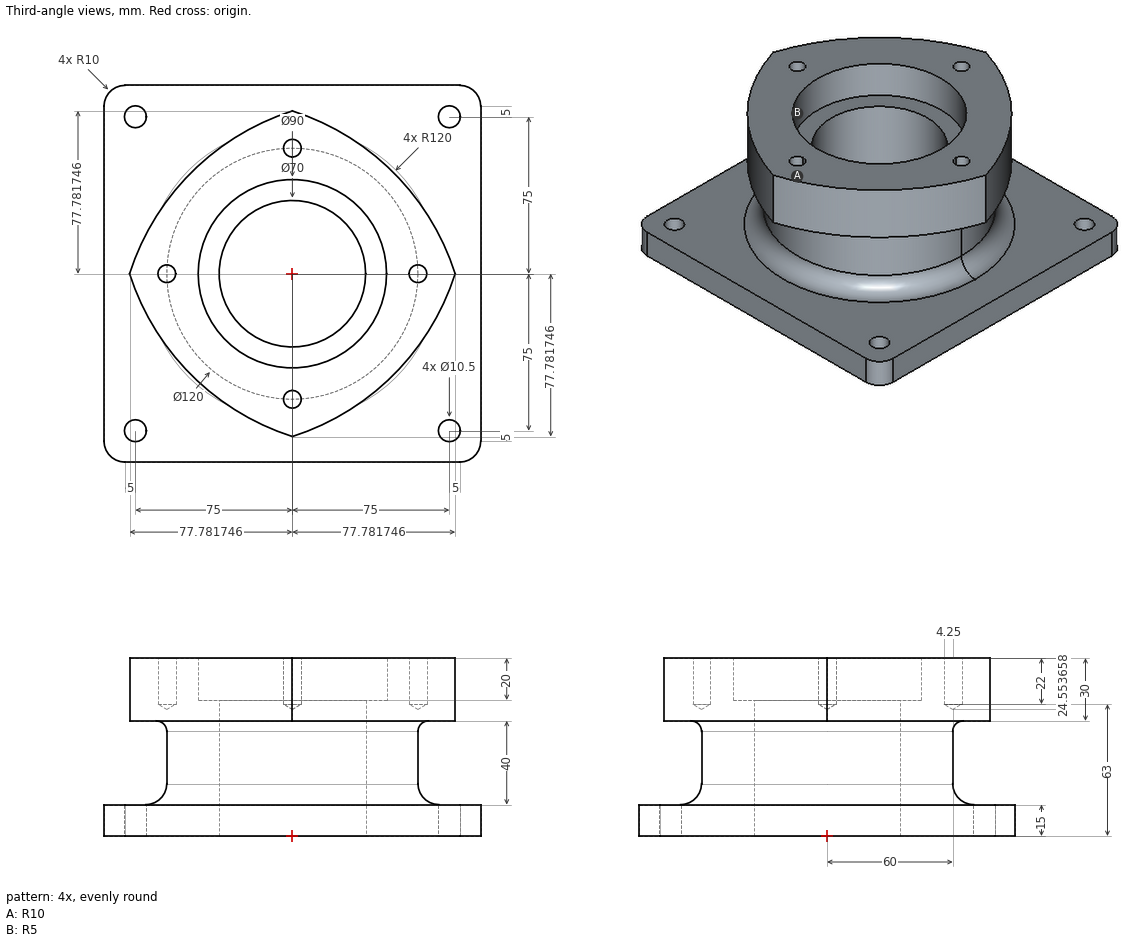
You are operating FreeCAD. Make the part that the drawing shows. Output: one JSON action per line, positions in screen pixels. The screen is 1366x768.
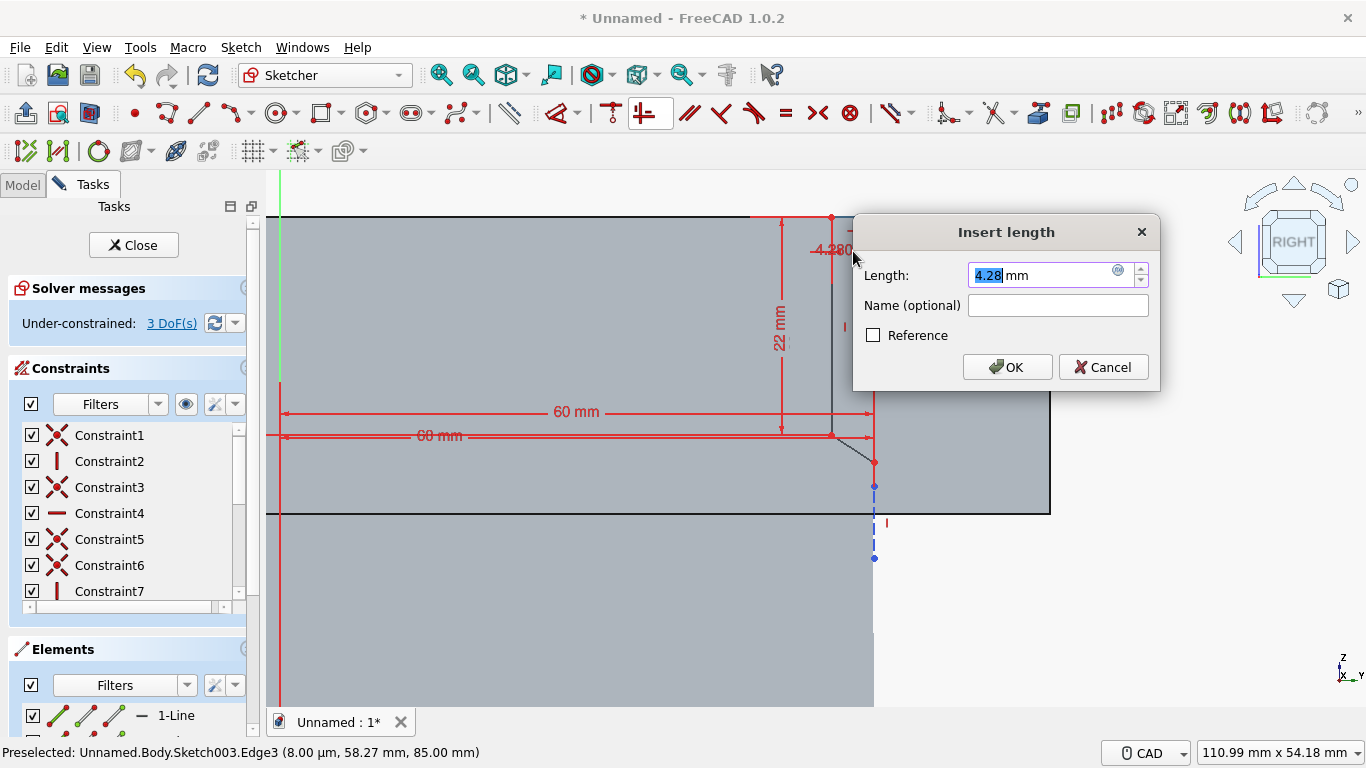
{"action": "type", "text": "4.25"}
{"action": "key", "text": "Return"}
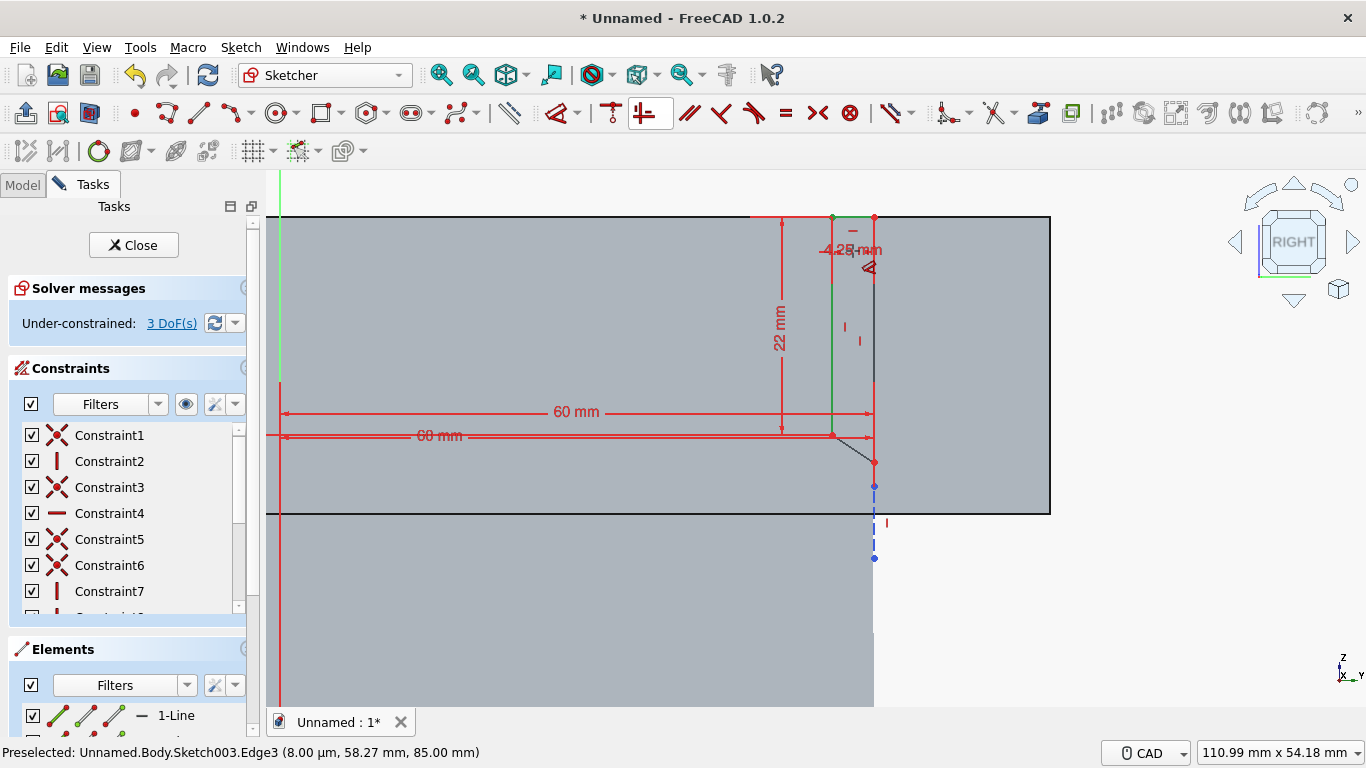
{"action": "left_click", "coordinate": [874, 389]}
{"action": "left_click", "coordinate": [908, 340]}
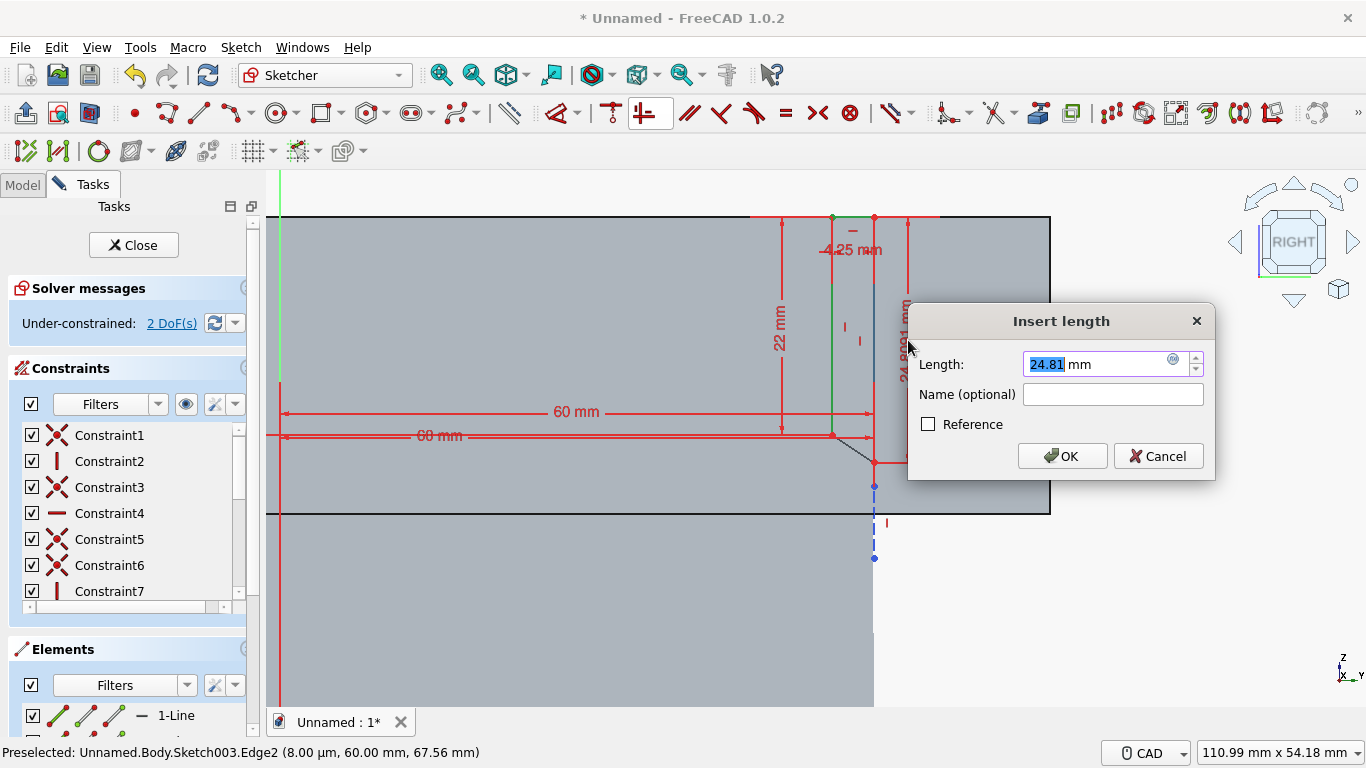
{"action": "type", "text": "24.553658"}
{"action": "key", "text": "Return"}
{"action": "key", "text": "Escape"}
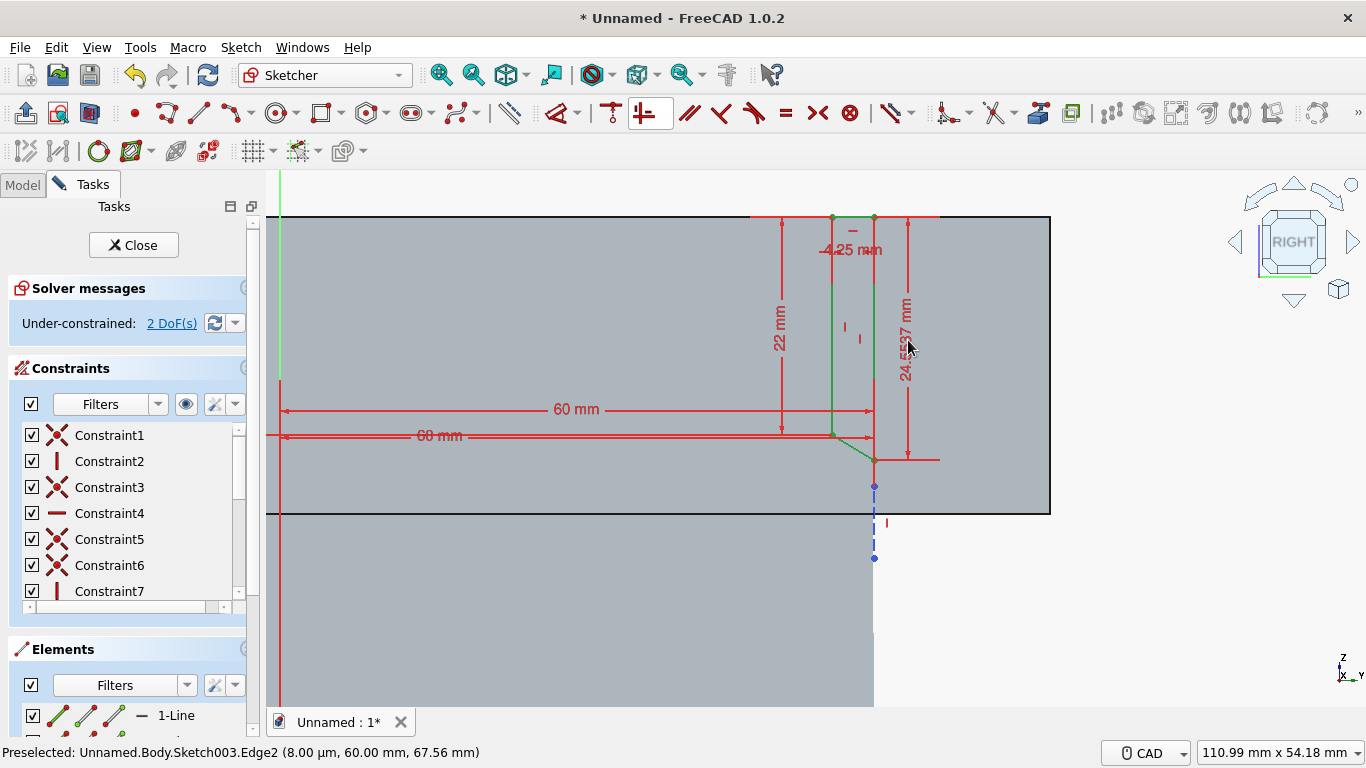
{"action": "left_click", "coordinate": [134, 245]}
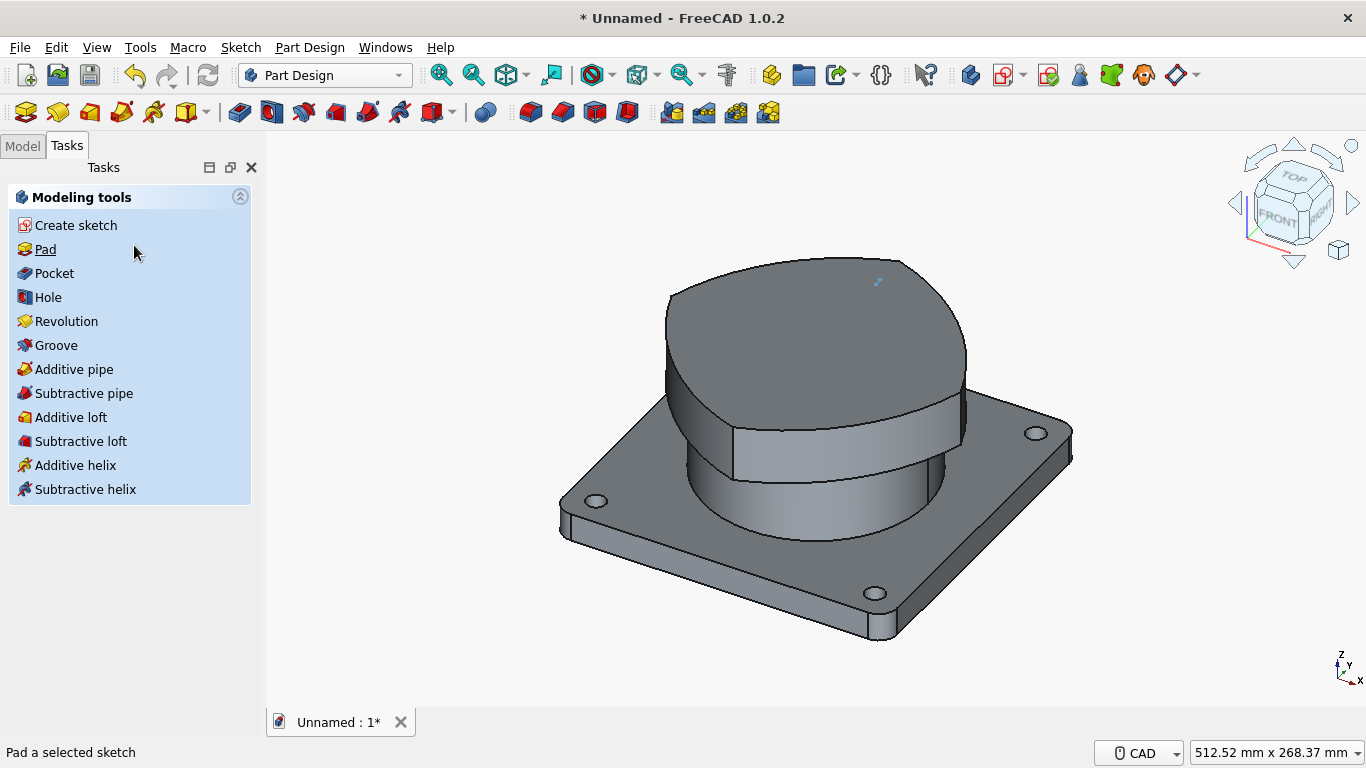
{"action": "left_click", "coordinate": [304, 112]}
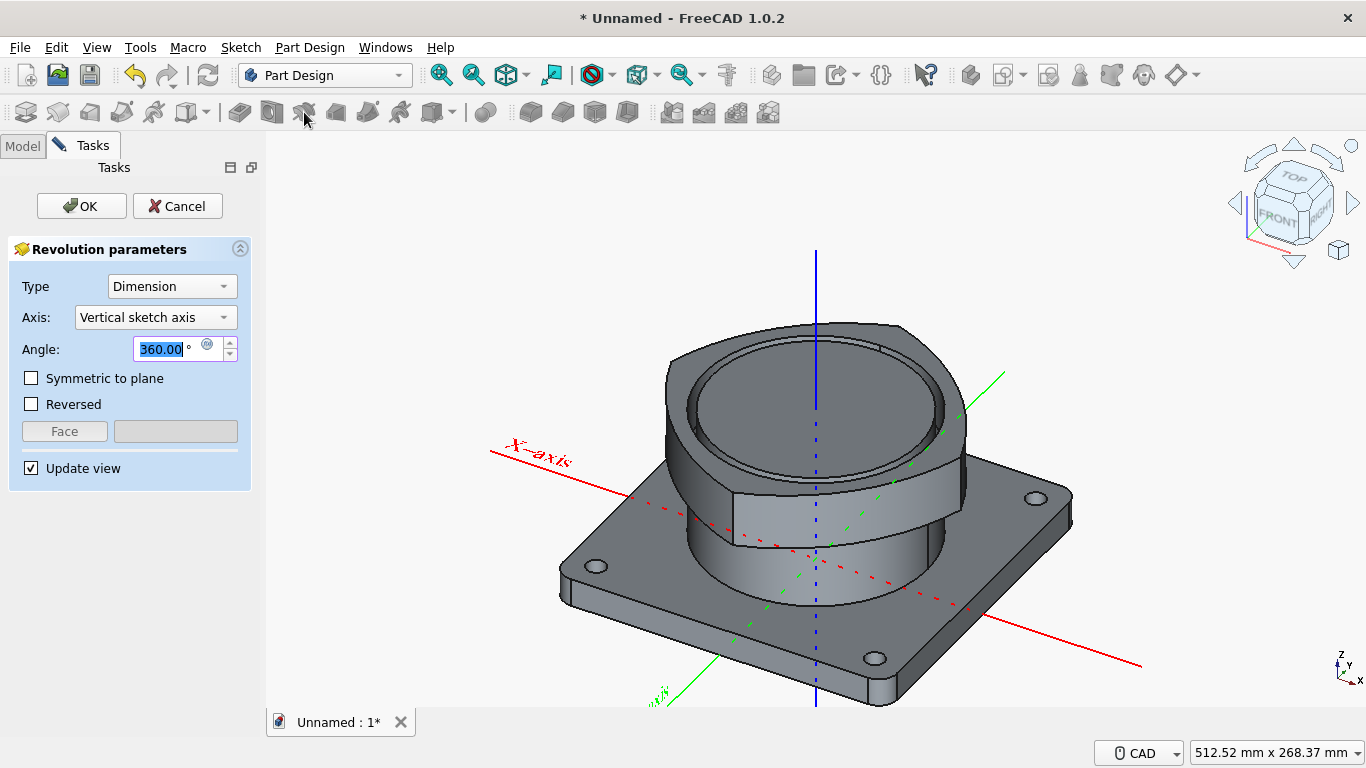
{"action": "left_click", "coordinate": [156, 318]}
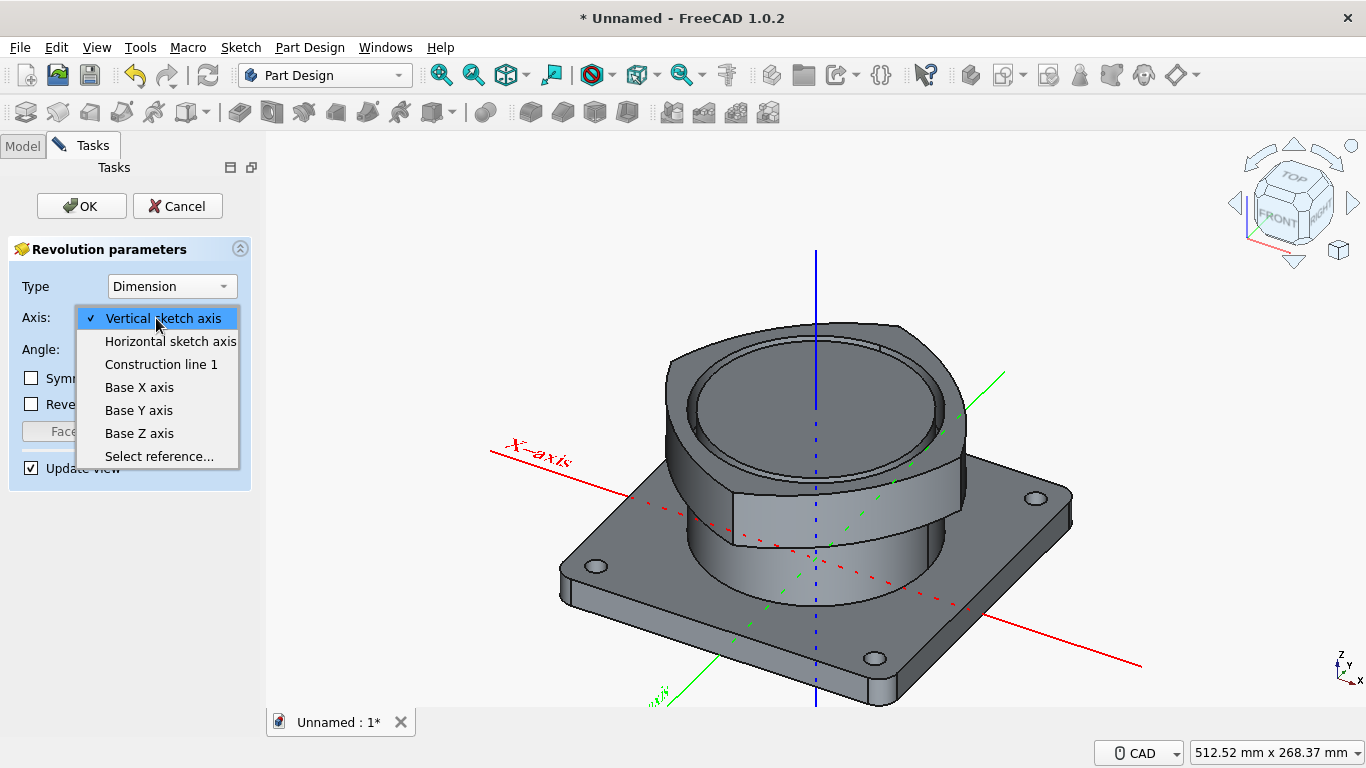
{"action": "left_click", "coordinate": [156, 364]}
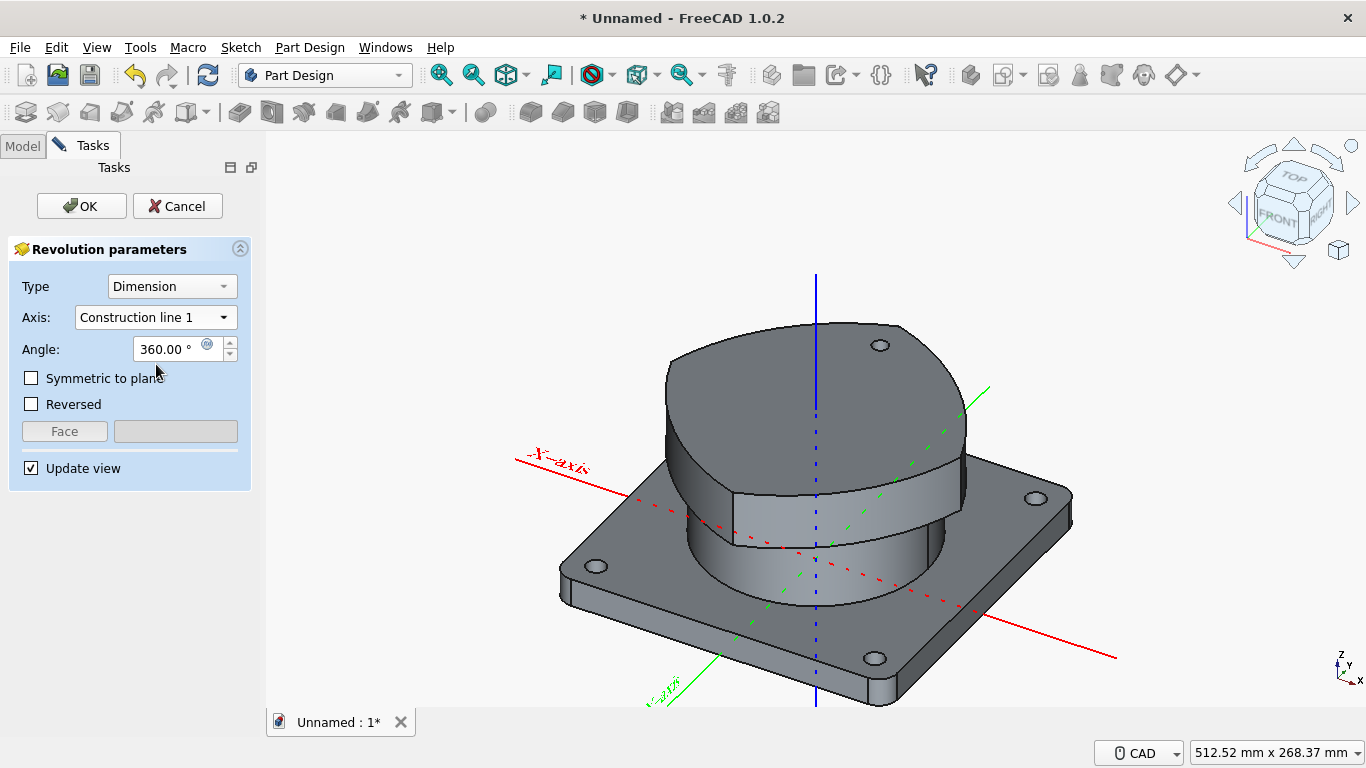
{"action": "left_click", "coordinate": [82, 206]}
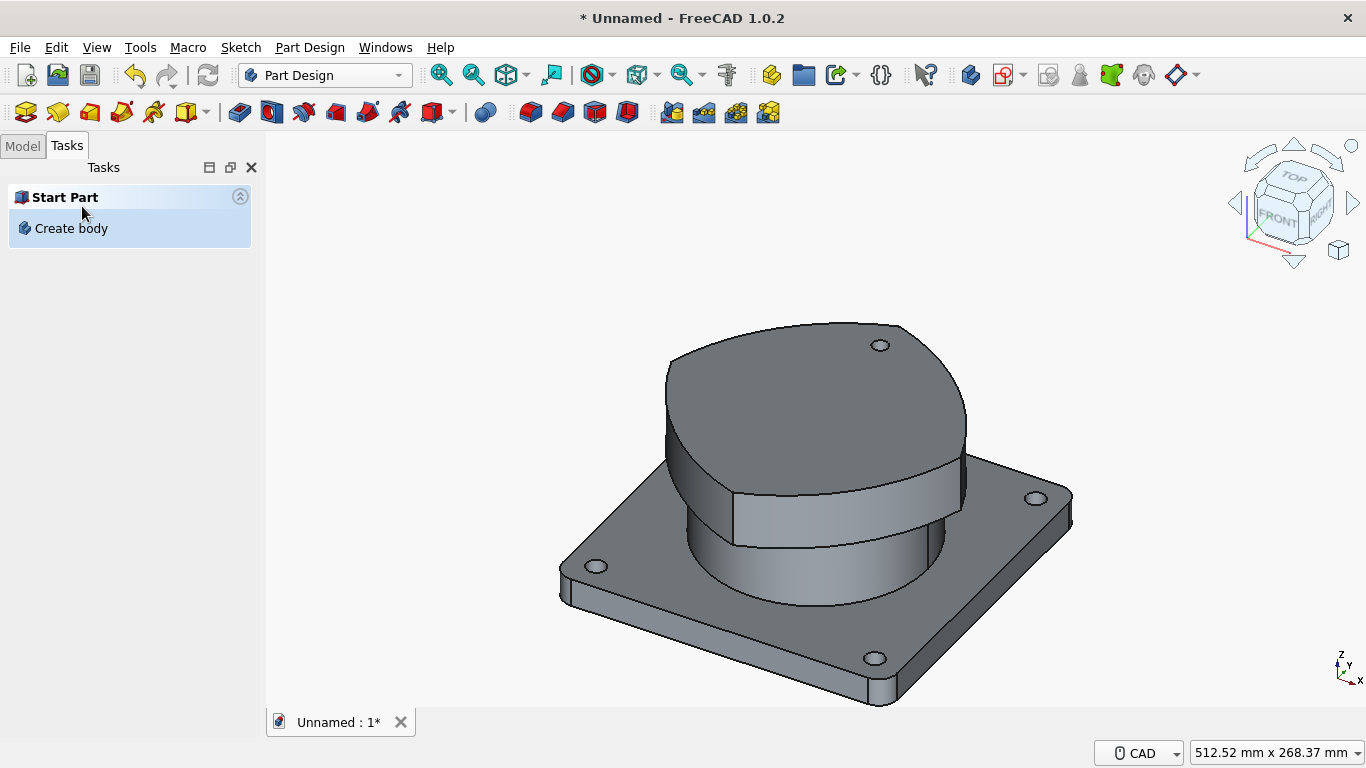
{"action": "left_click", "coordinate": [442, 76]}